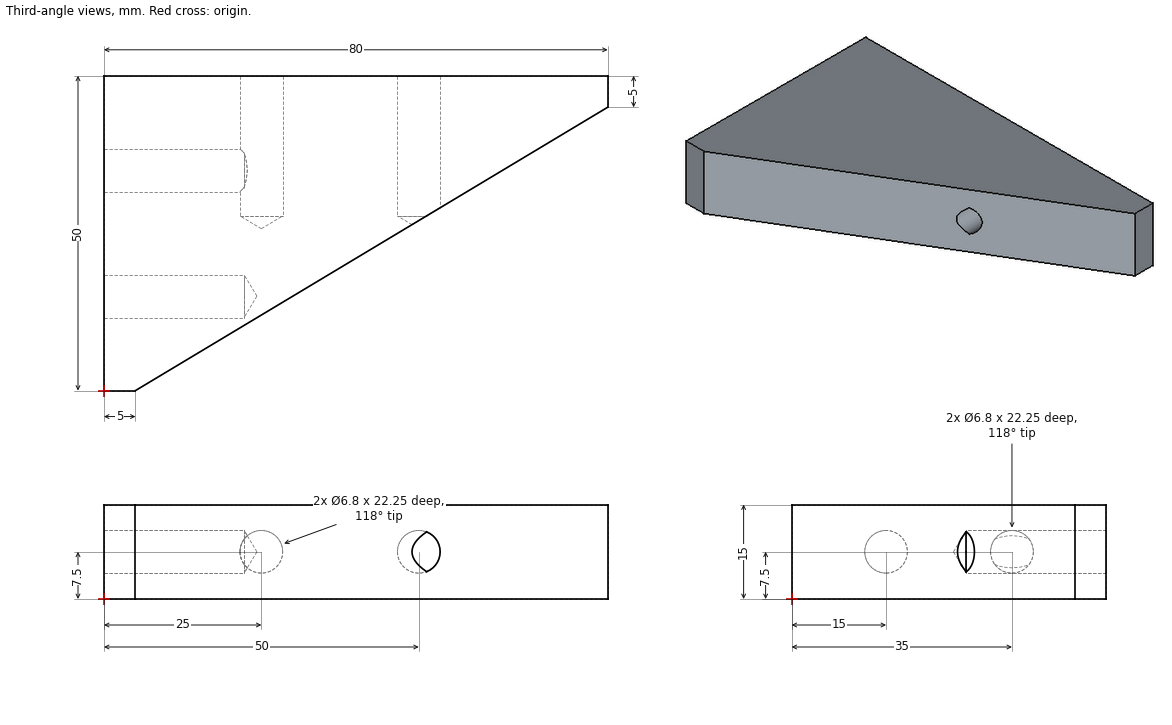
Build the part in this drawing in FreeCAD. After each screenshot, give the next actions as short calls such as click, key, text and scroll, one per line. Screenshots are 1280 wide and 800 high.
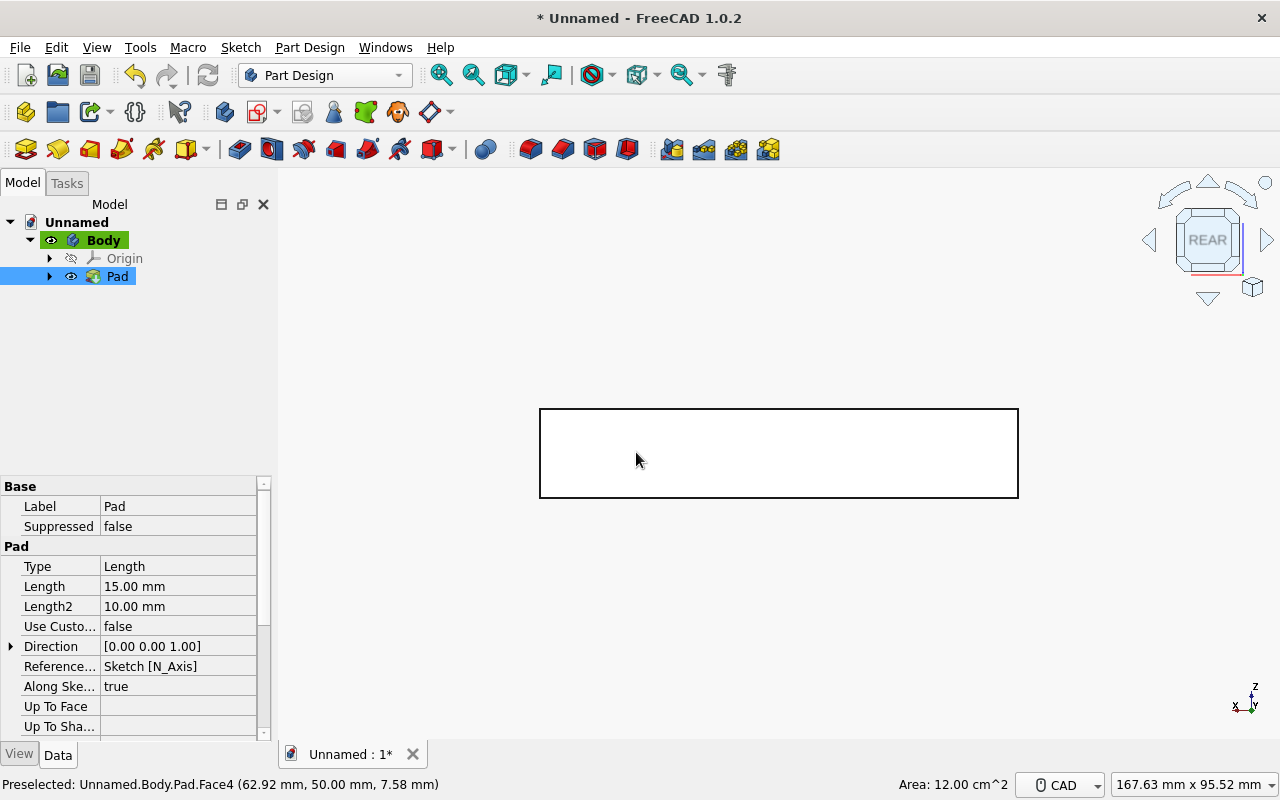
click(258, 112)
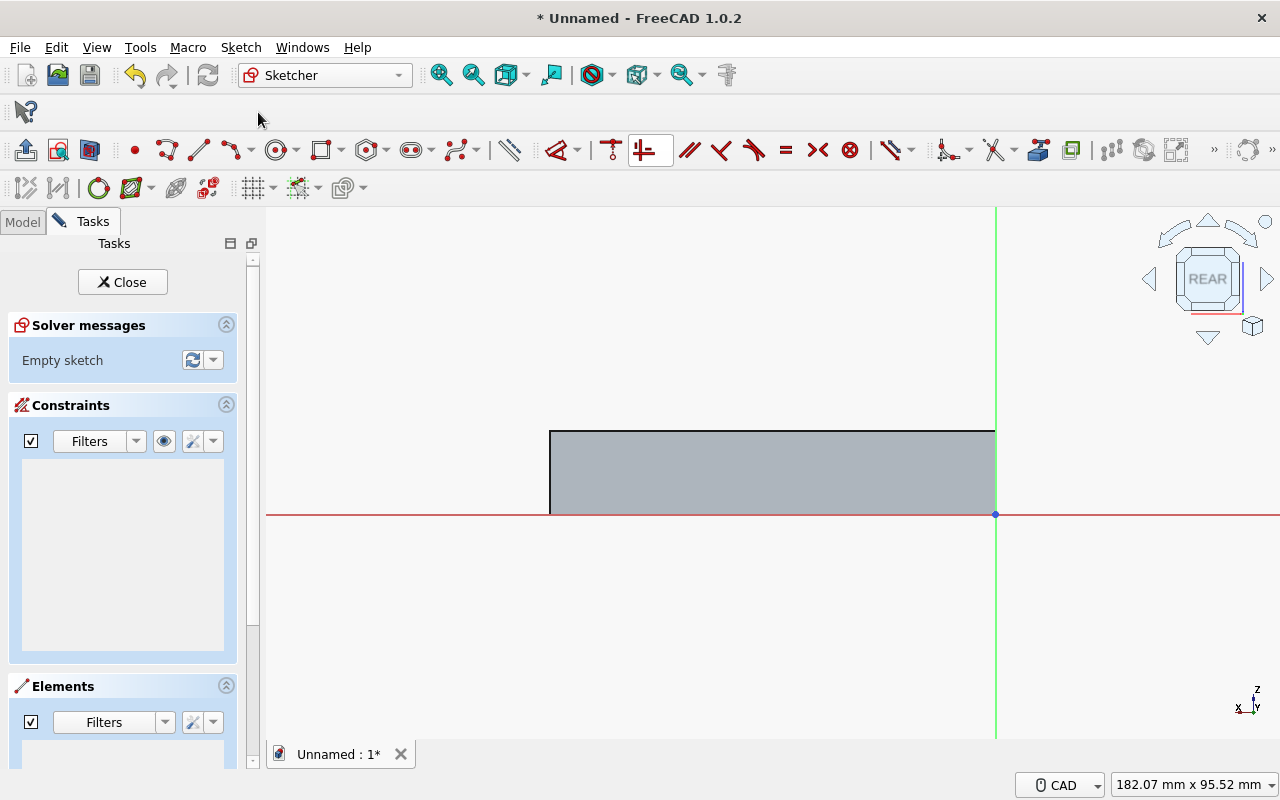
scroll(1020, 498, up, 3)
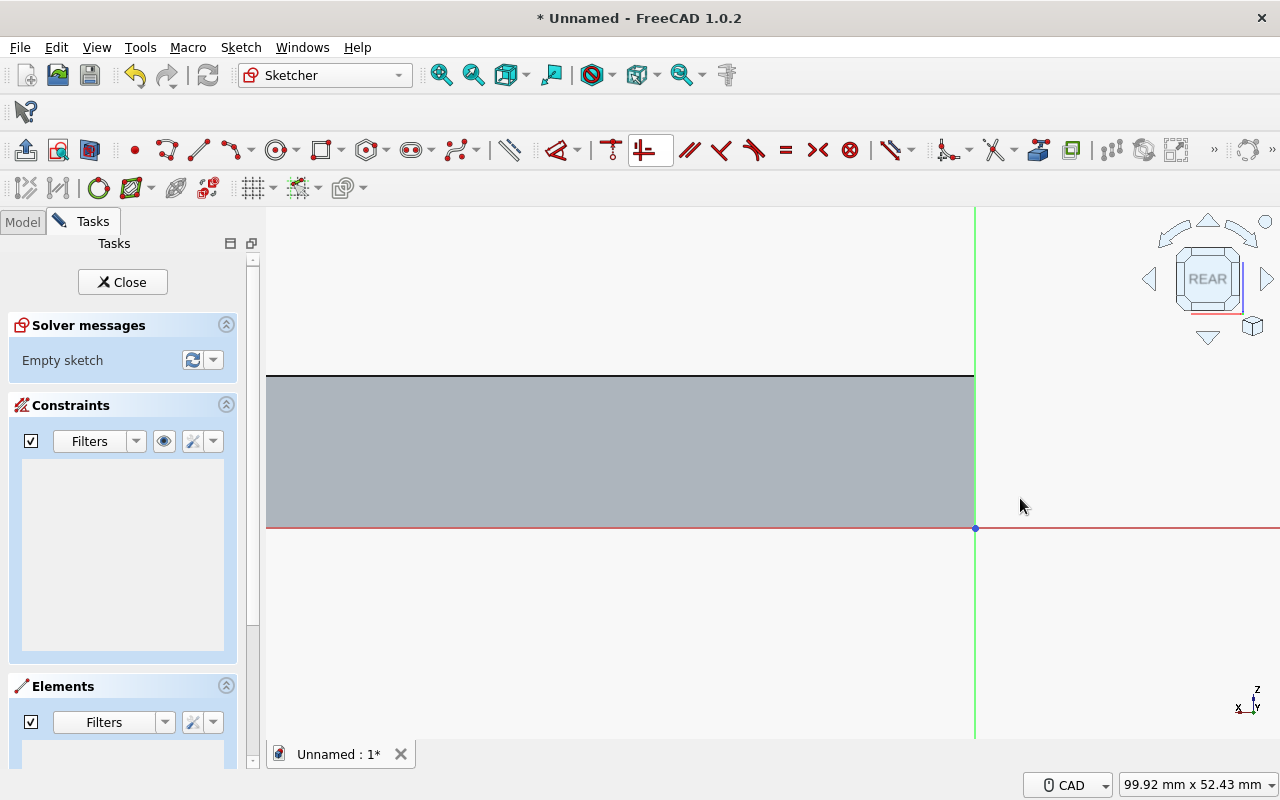
click(276, 150)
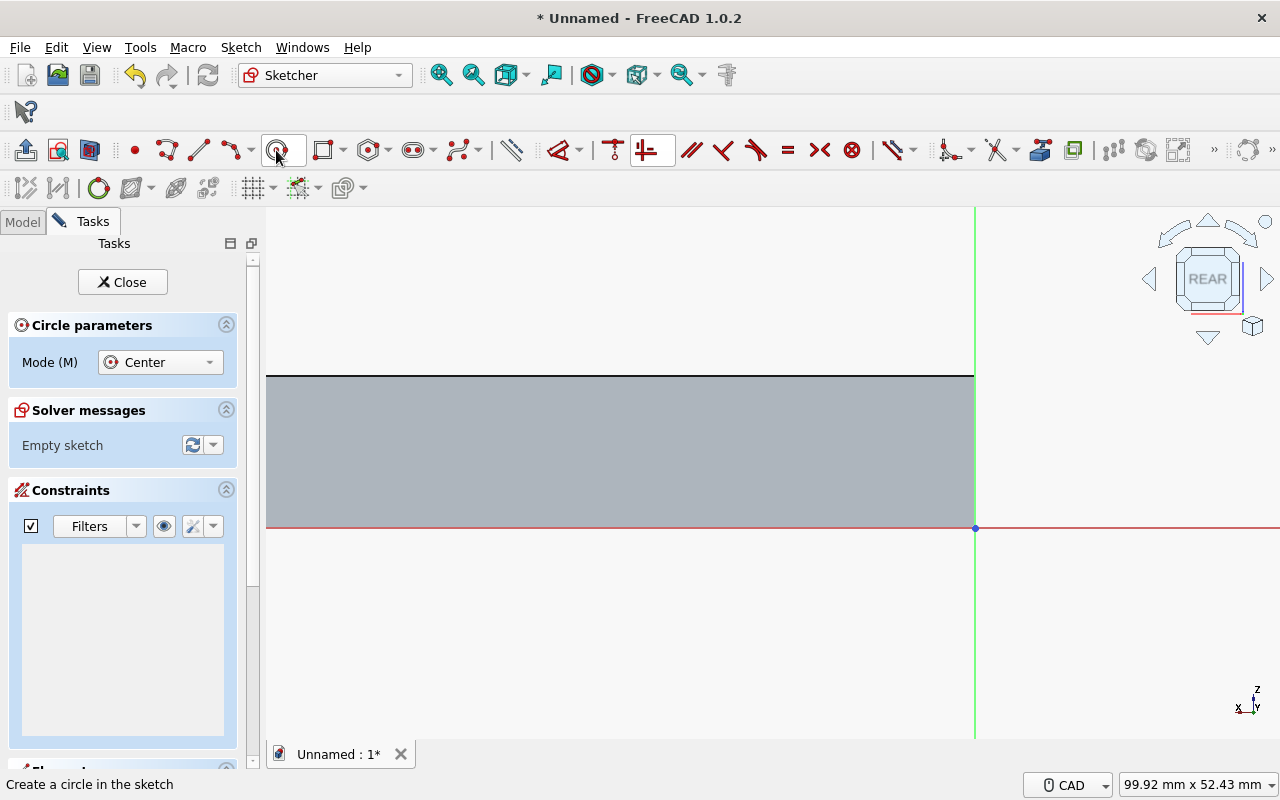
click(722, 452)
move(746, 428)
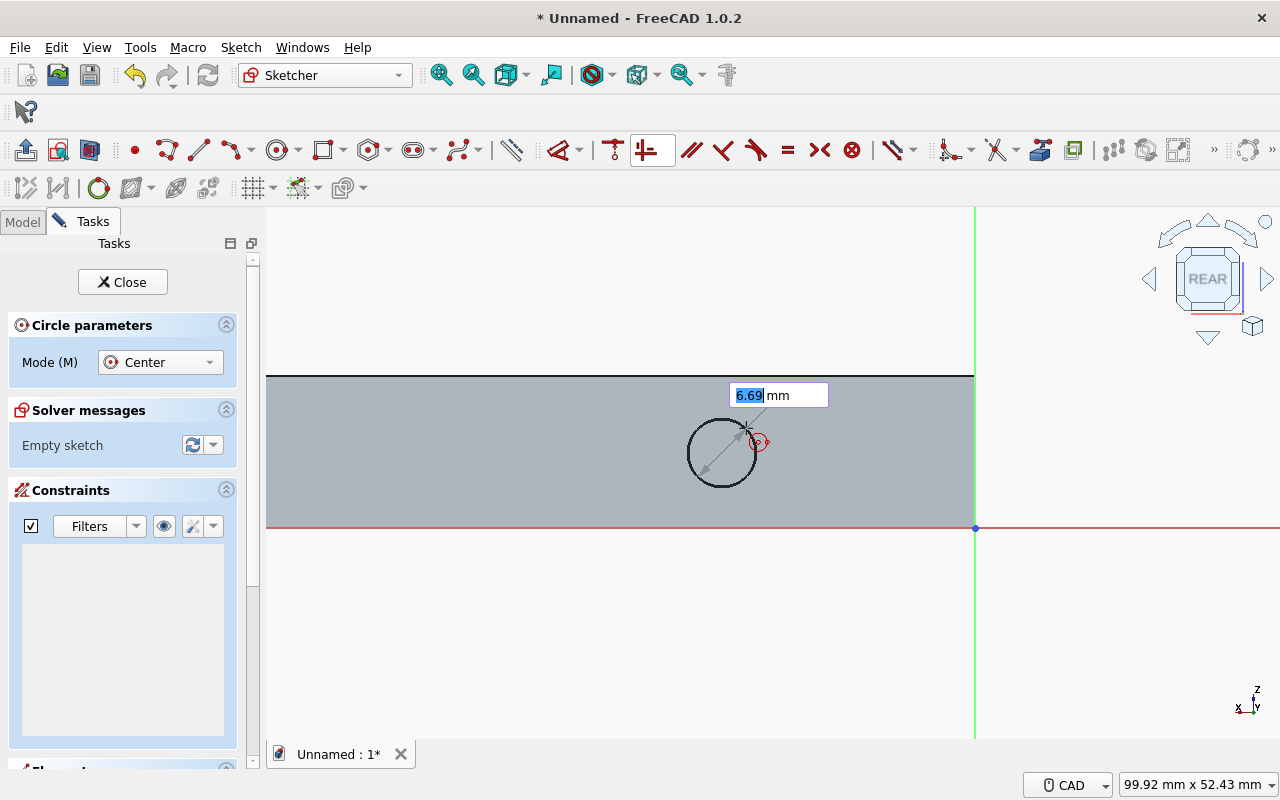
text(6.8)
key(Return)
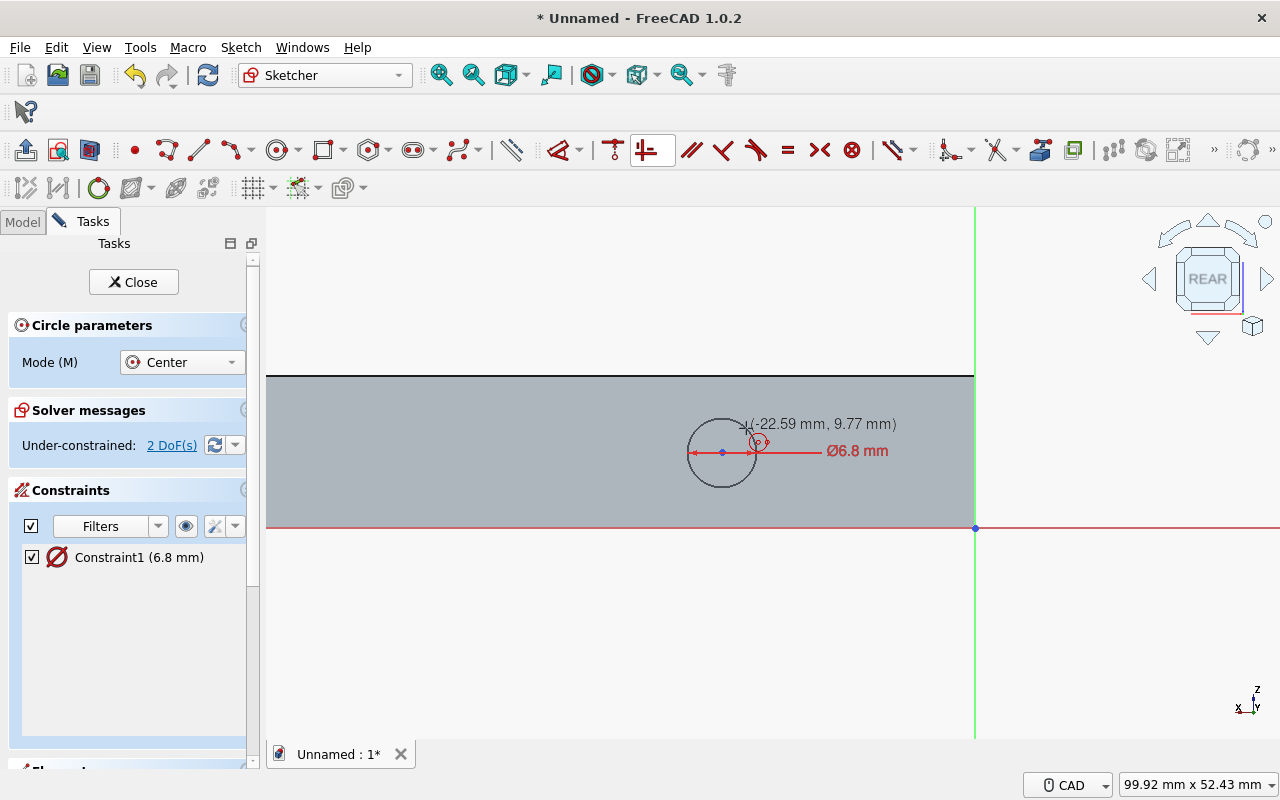
click(468, 452)
move(492, 428)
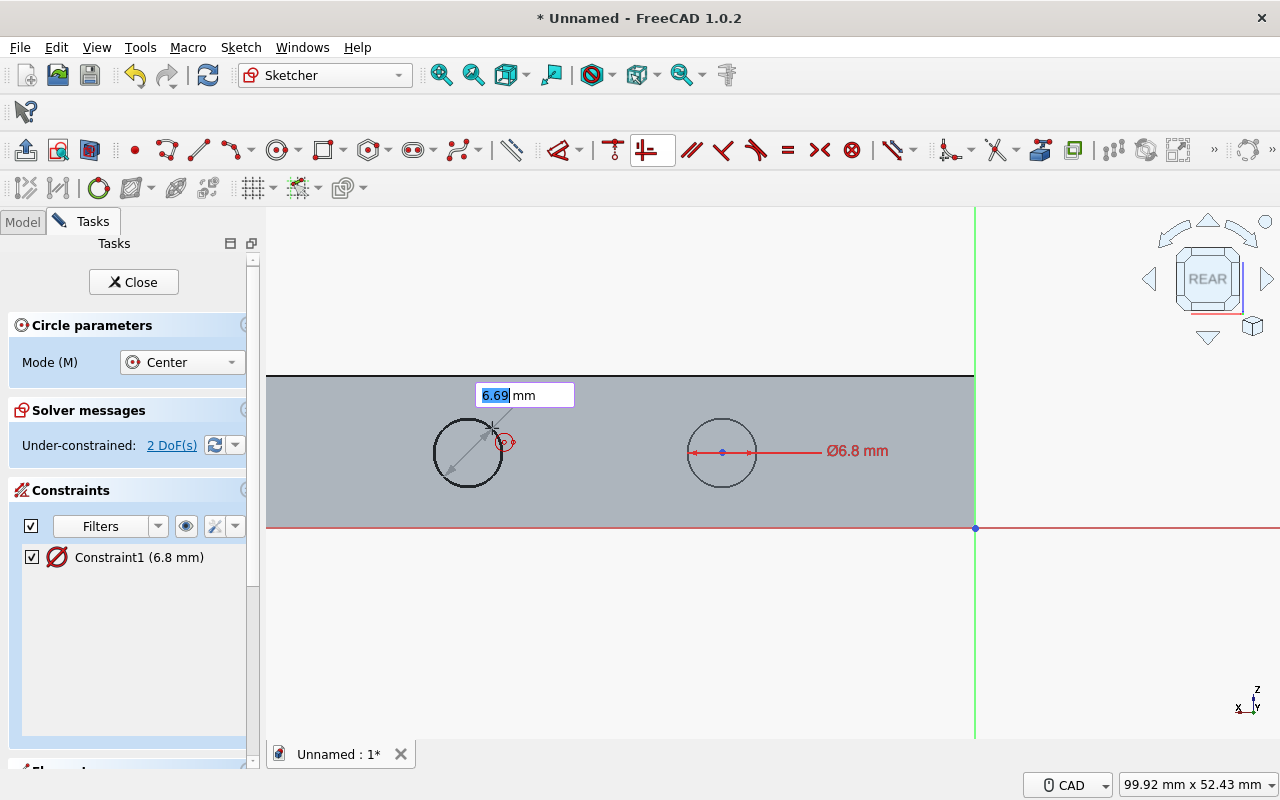
text(6.8)
key(Return)
key(Escape)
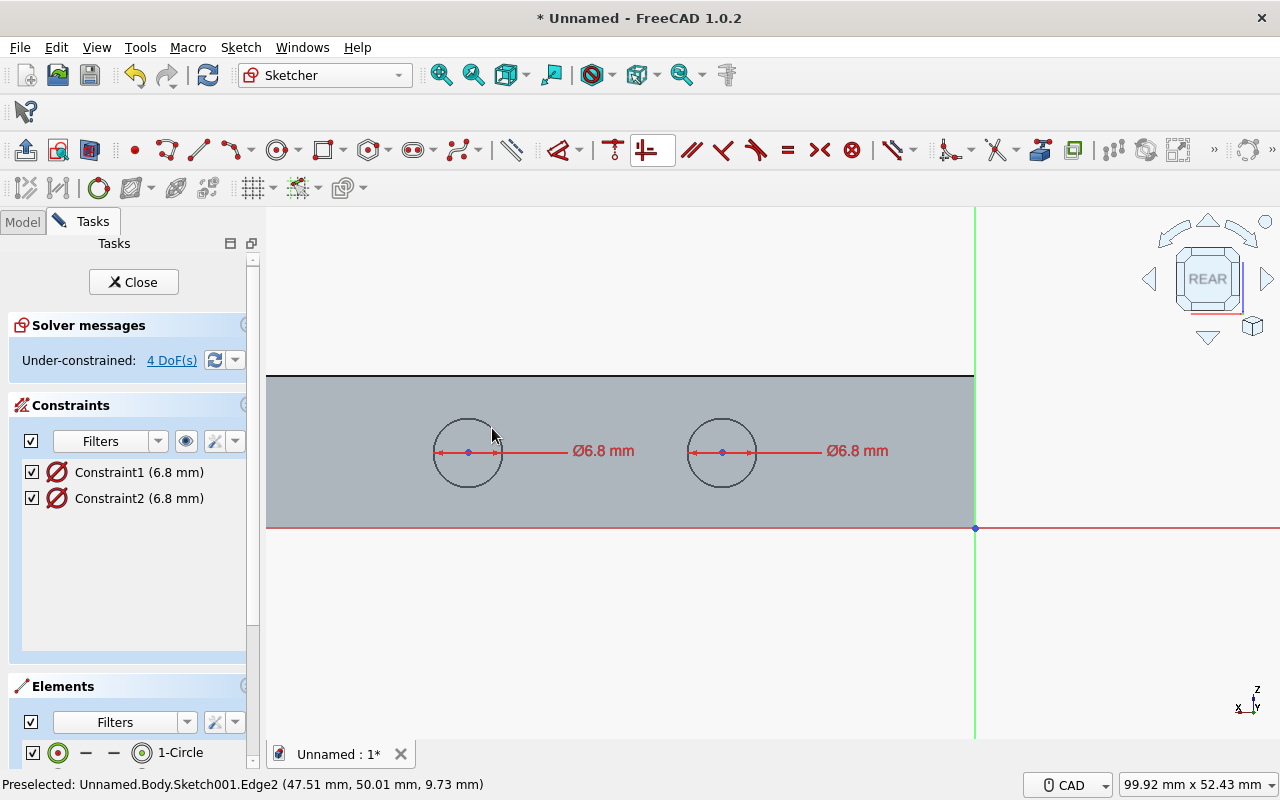
click(558, 150)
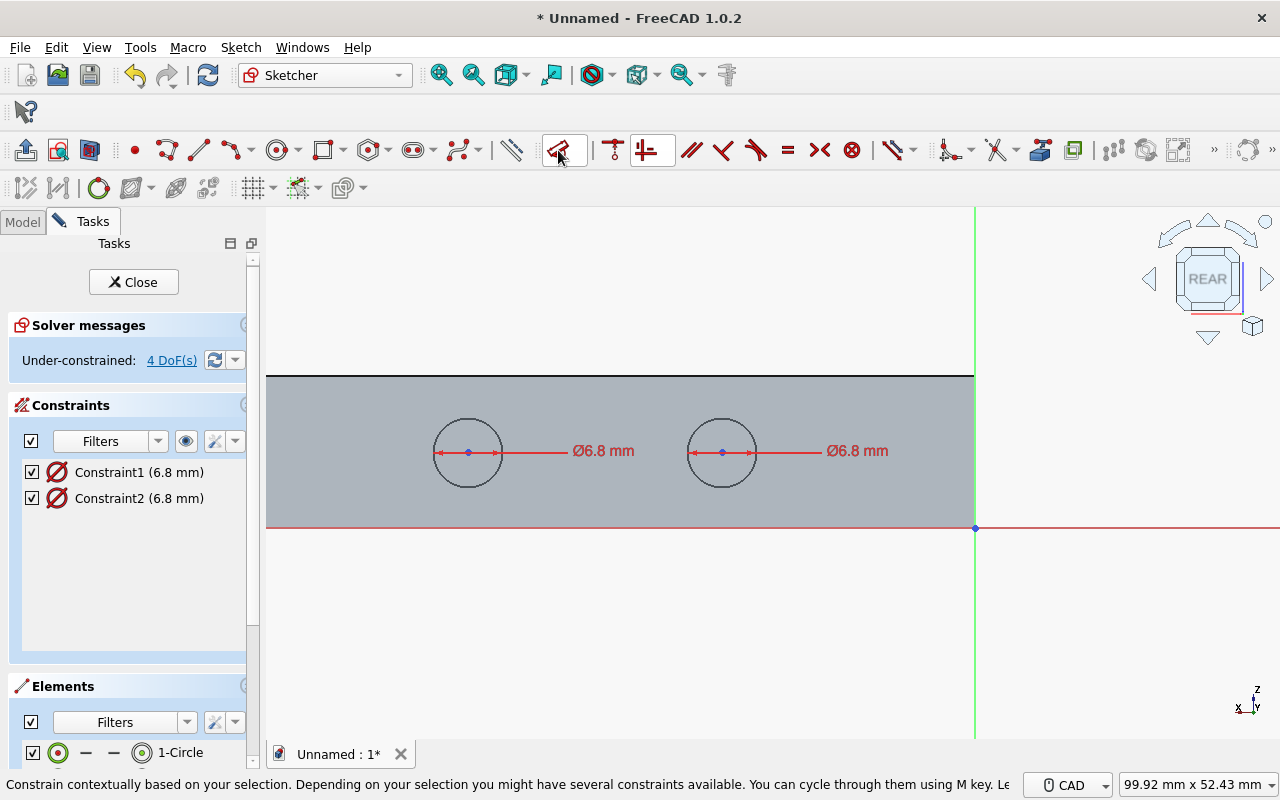
click(722, 453)
click(849, 562)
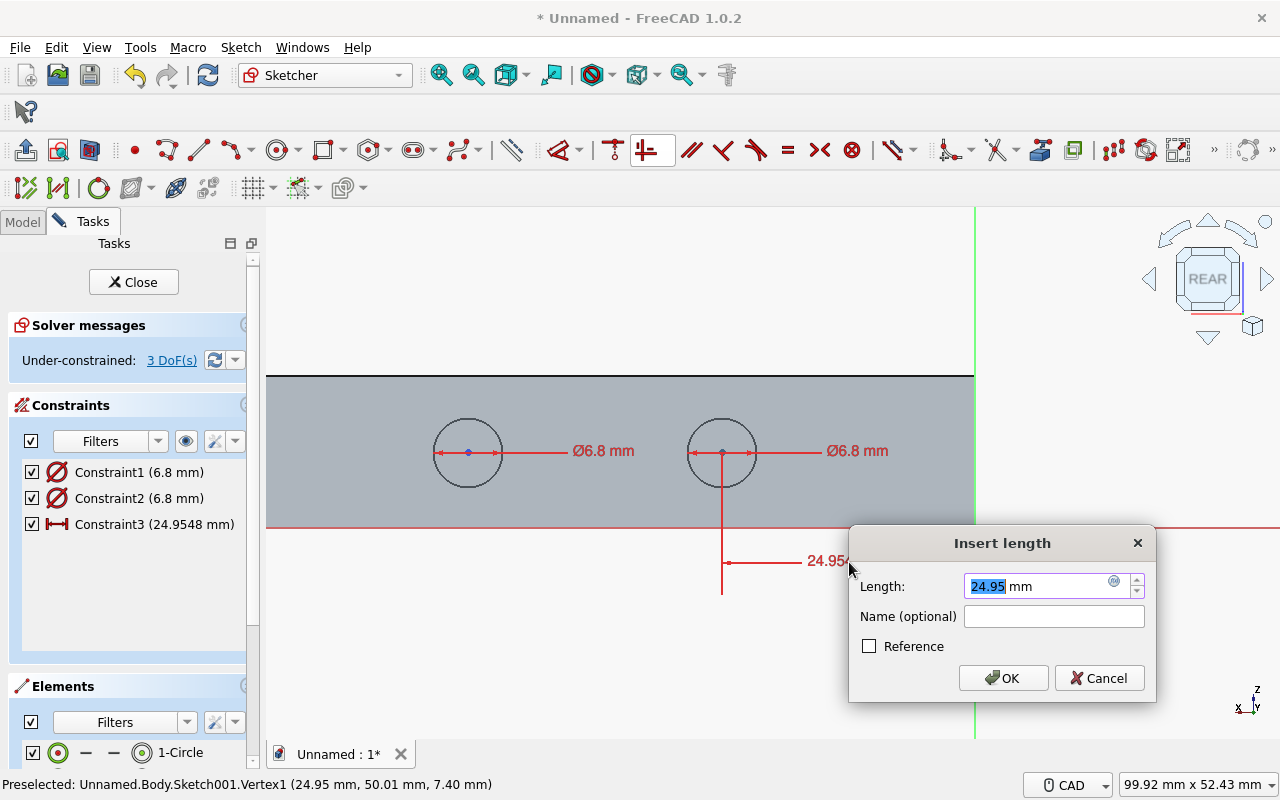
text(25)
key(Return)